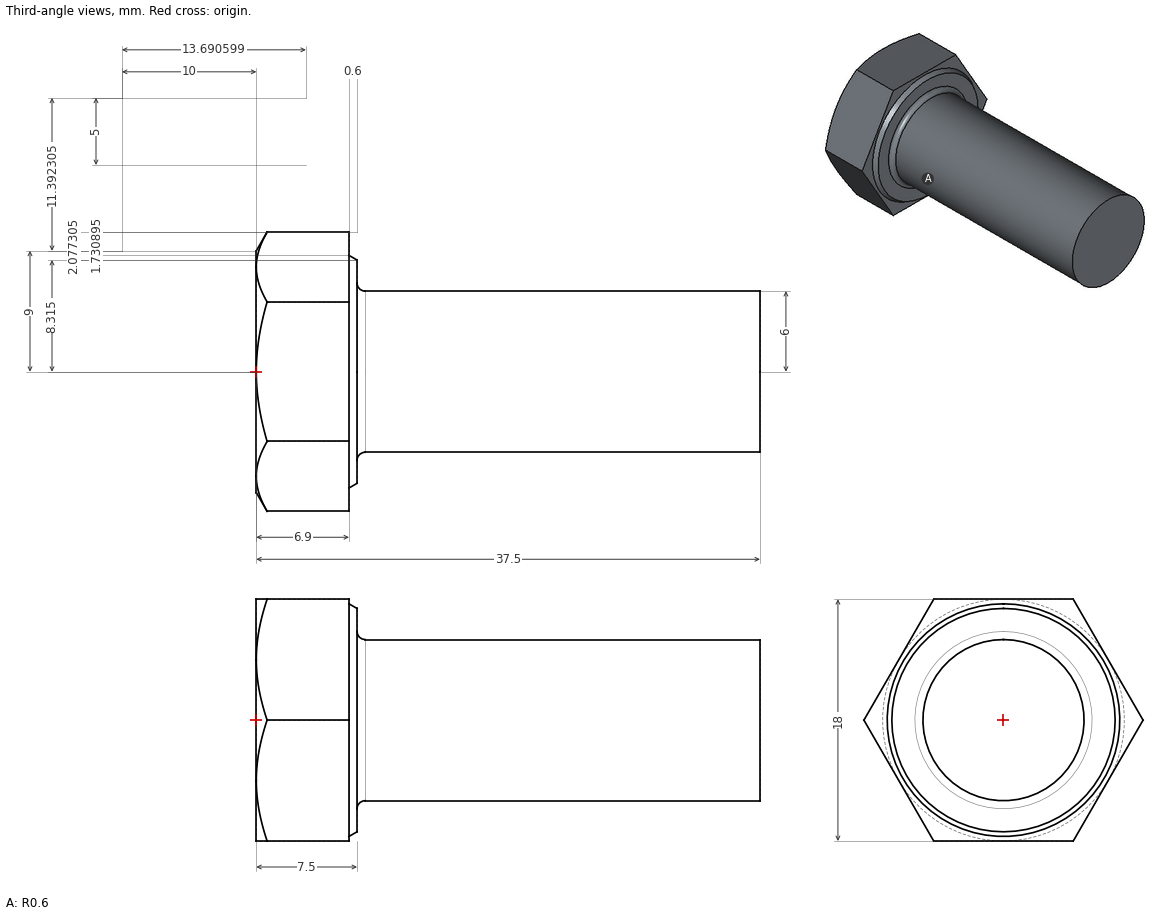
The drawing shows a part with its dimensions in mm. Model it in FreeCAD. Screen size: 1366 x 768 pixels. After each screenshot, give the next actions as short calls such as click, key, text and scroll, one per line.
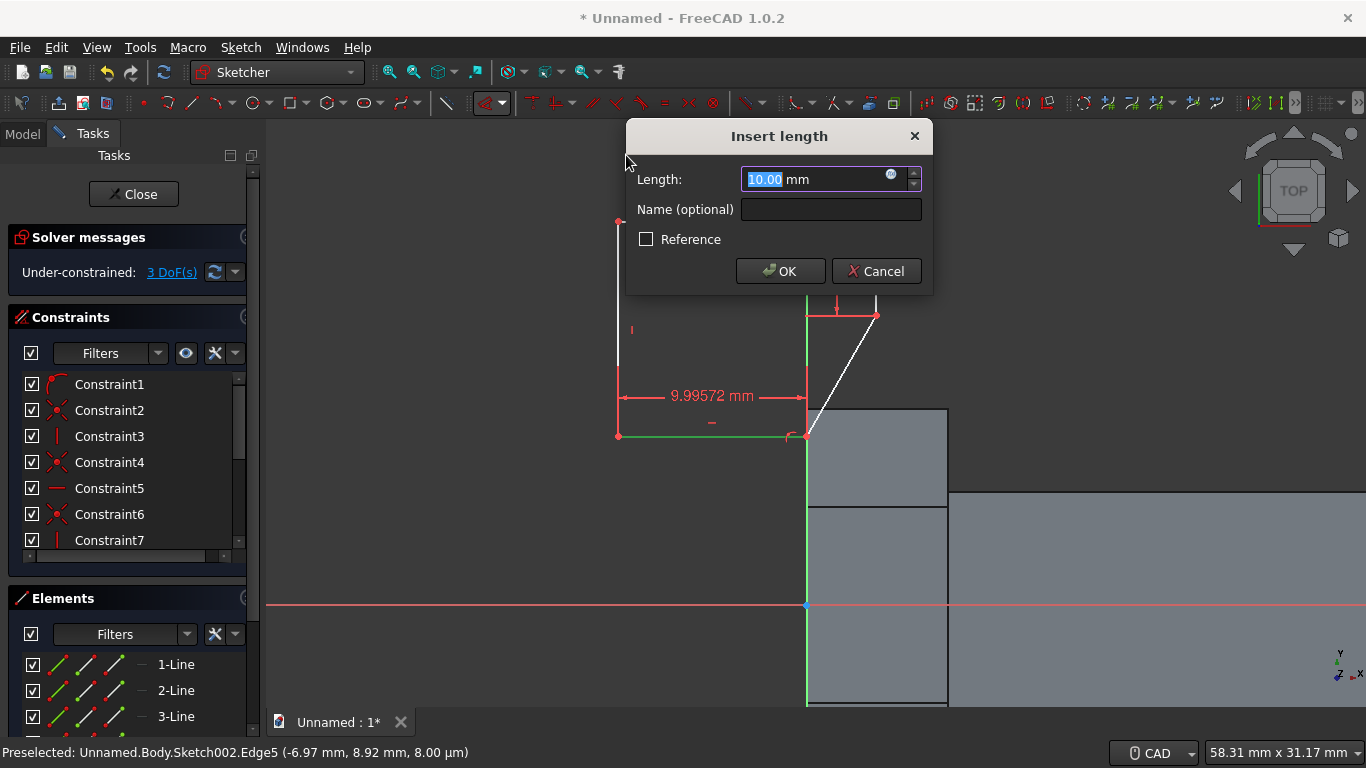
text(10)
key(Return)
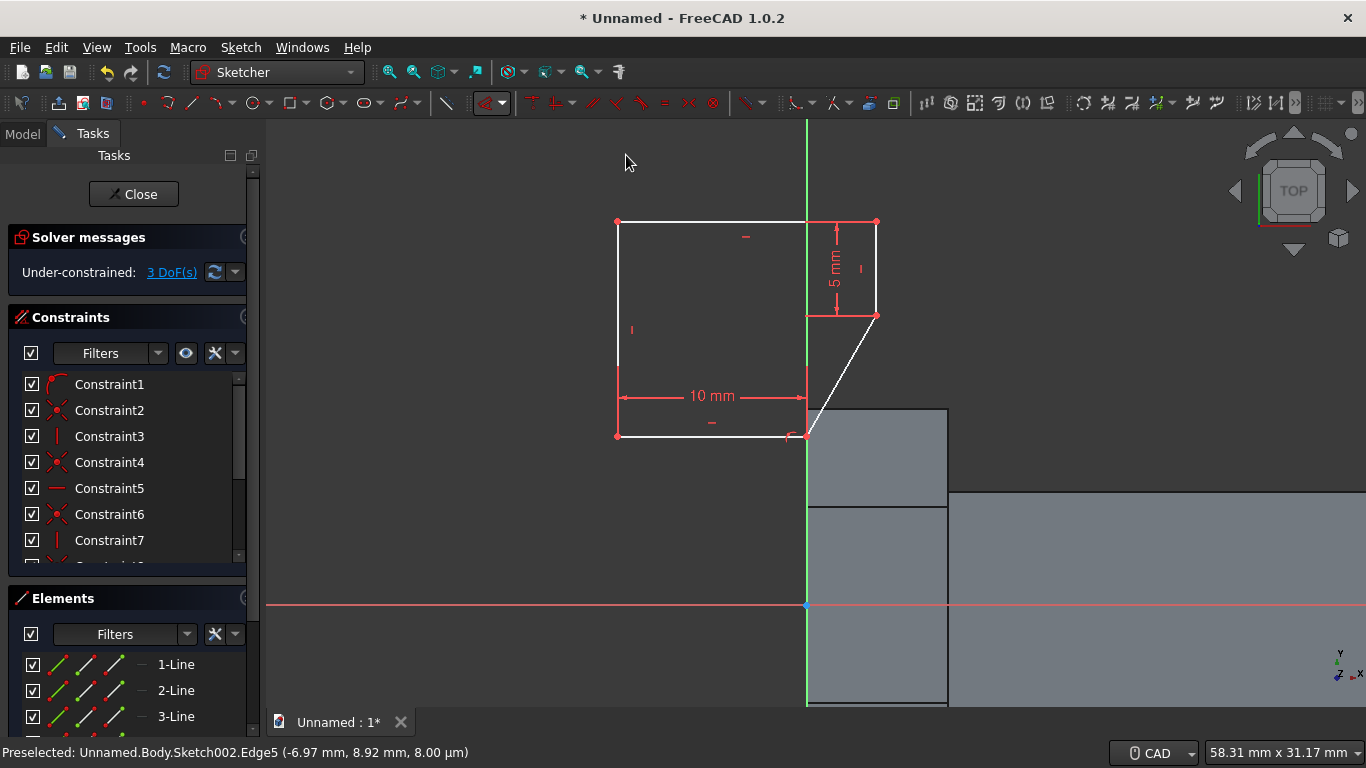
click(807, 437)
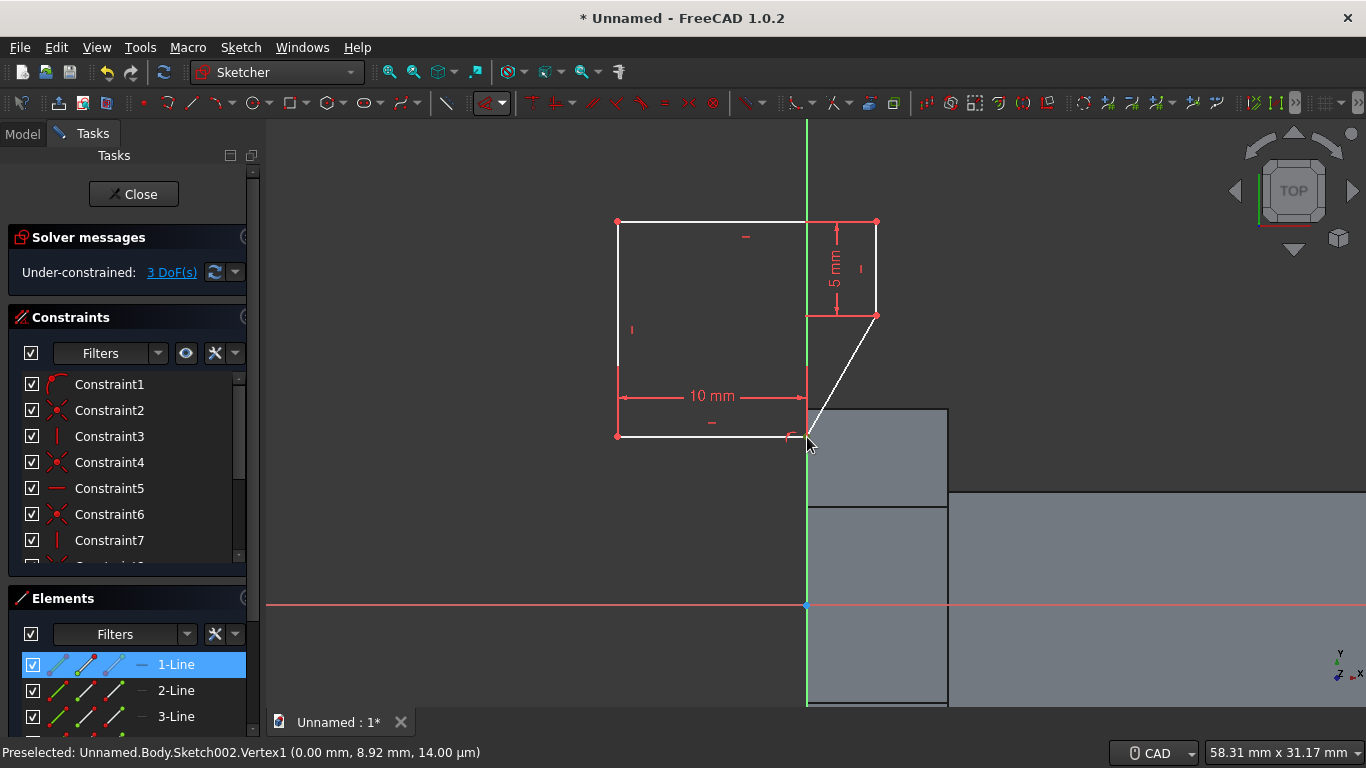
key(i)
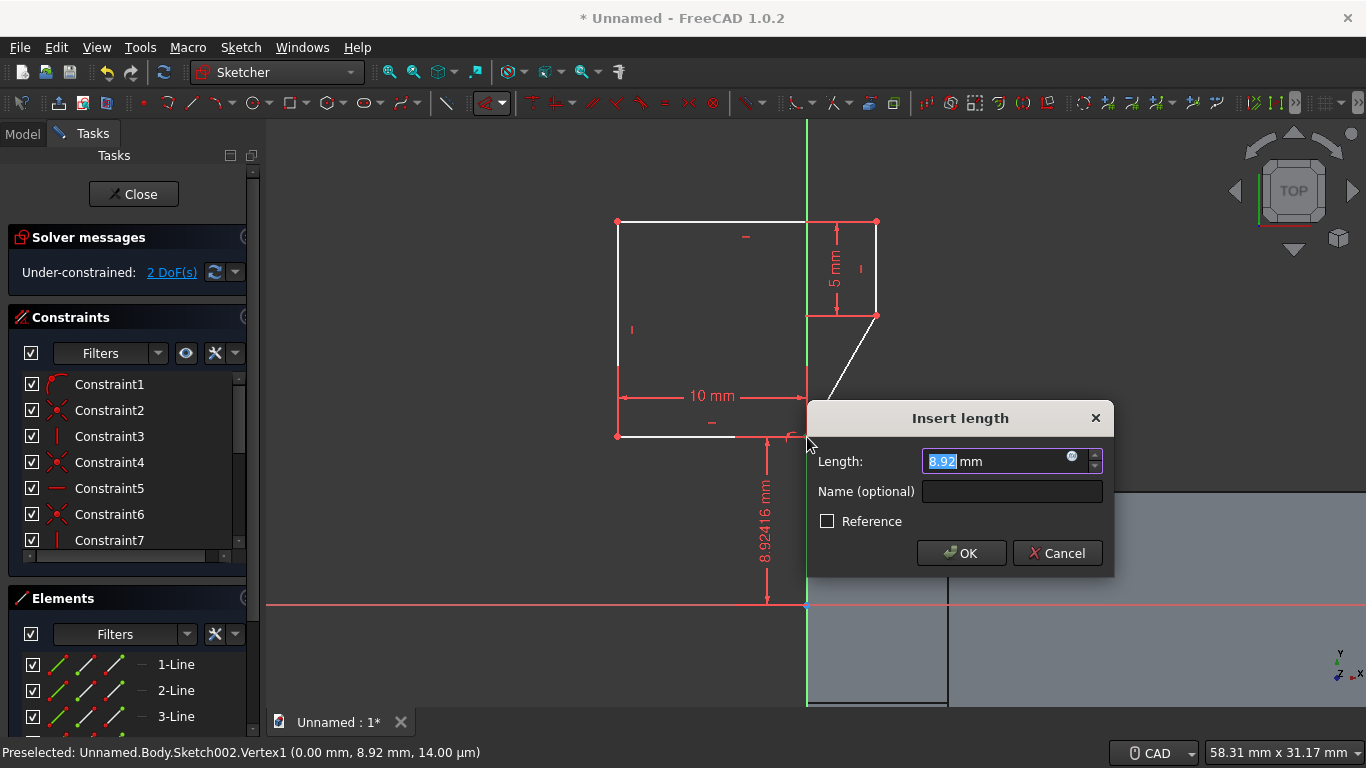
text(9)
key(Return)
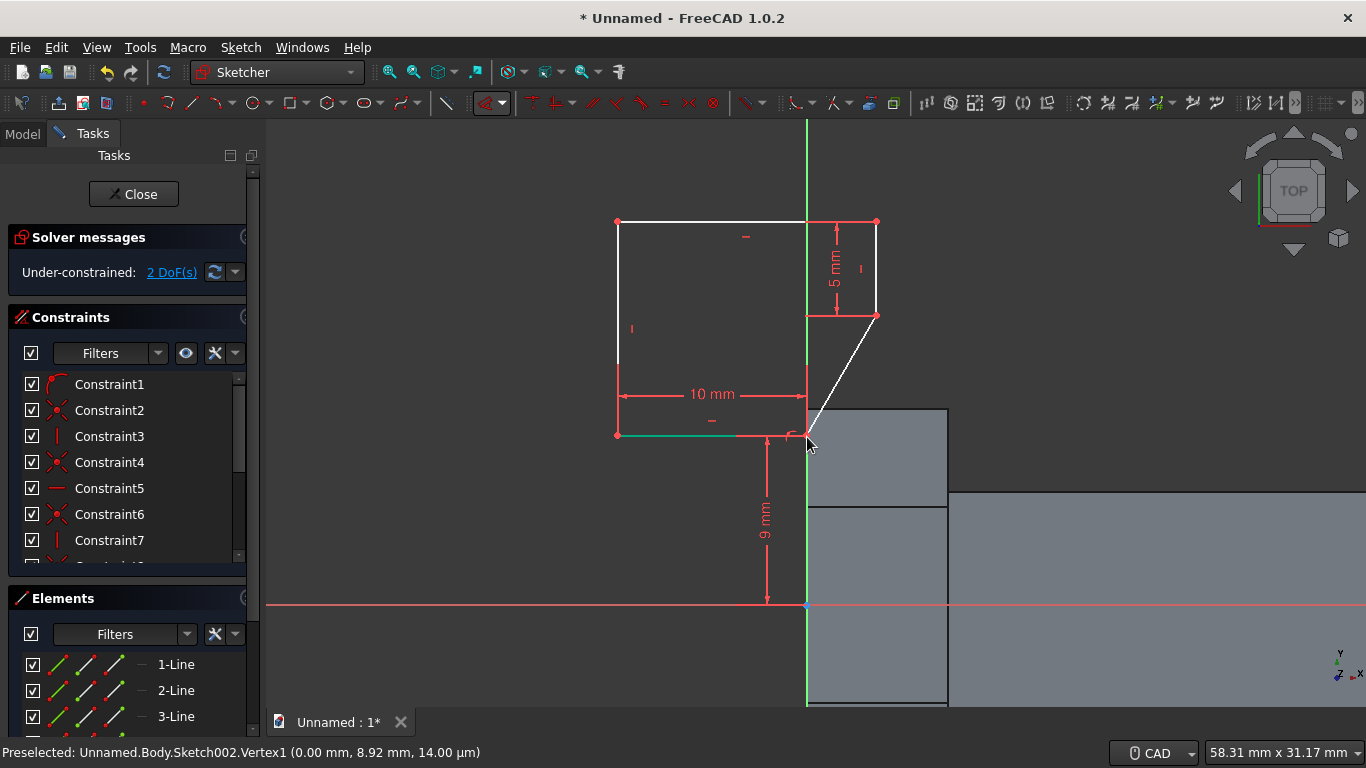
click(695, 222)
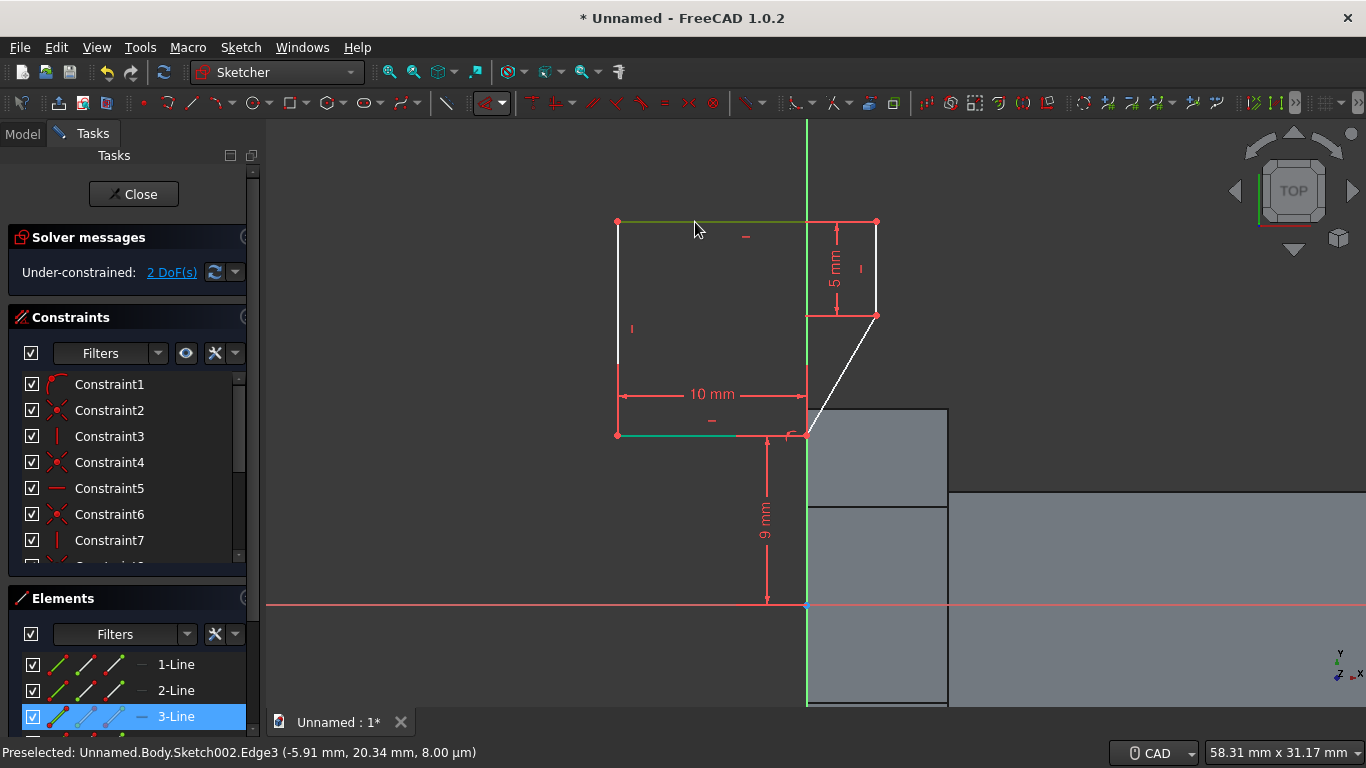
click(504, 104)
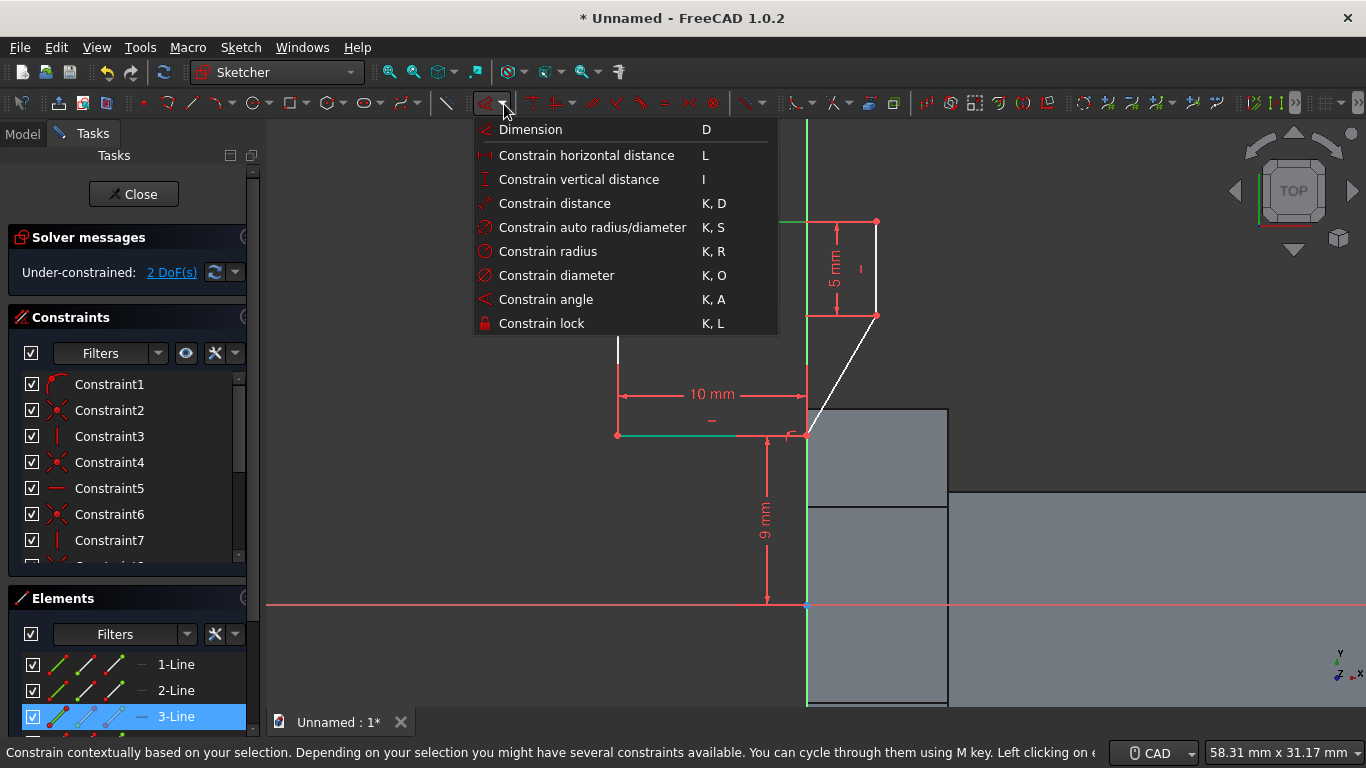
click(626, 155)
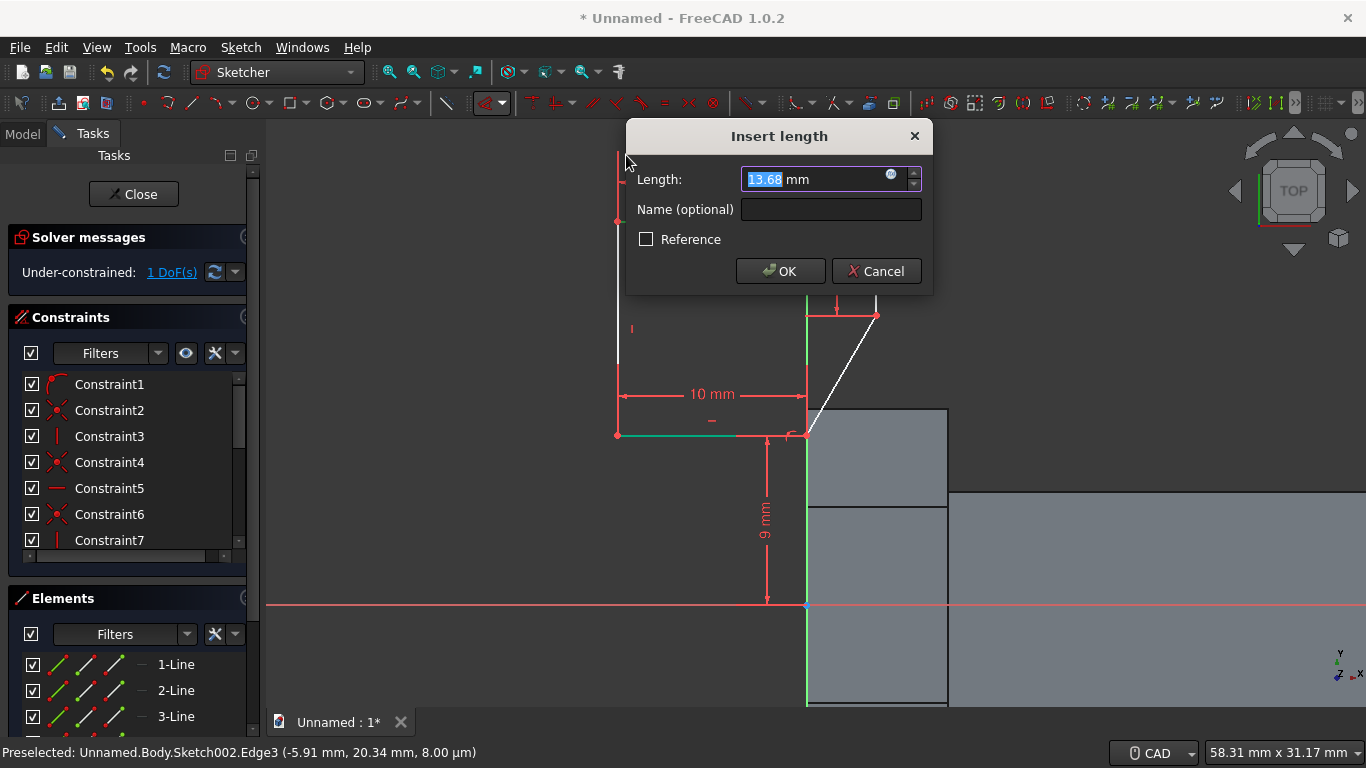
text(13.690599)
key(Return)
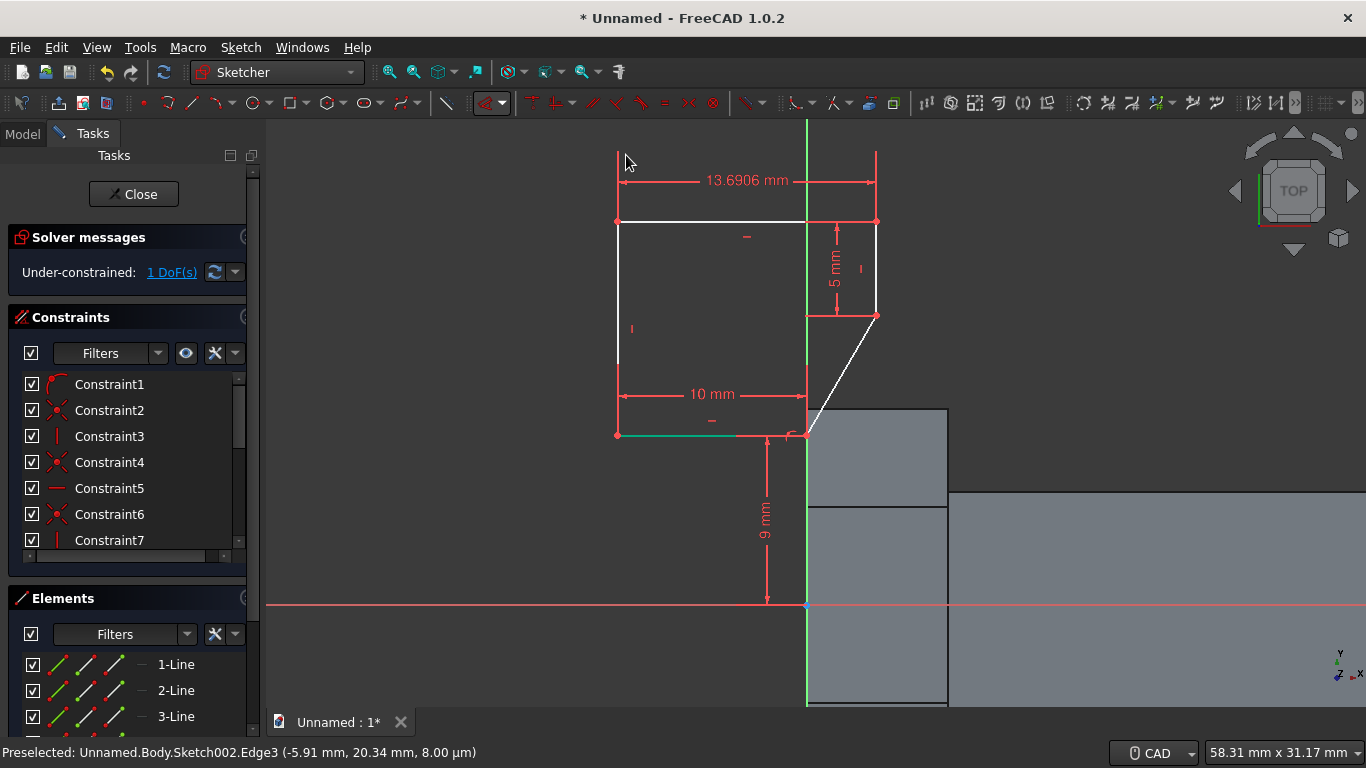
click(618, 286)